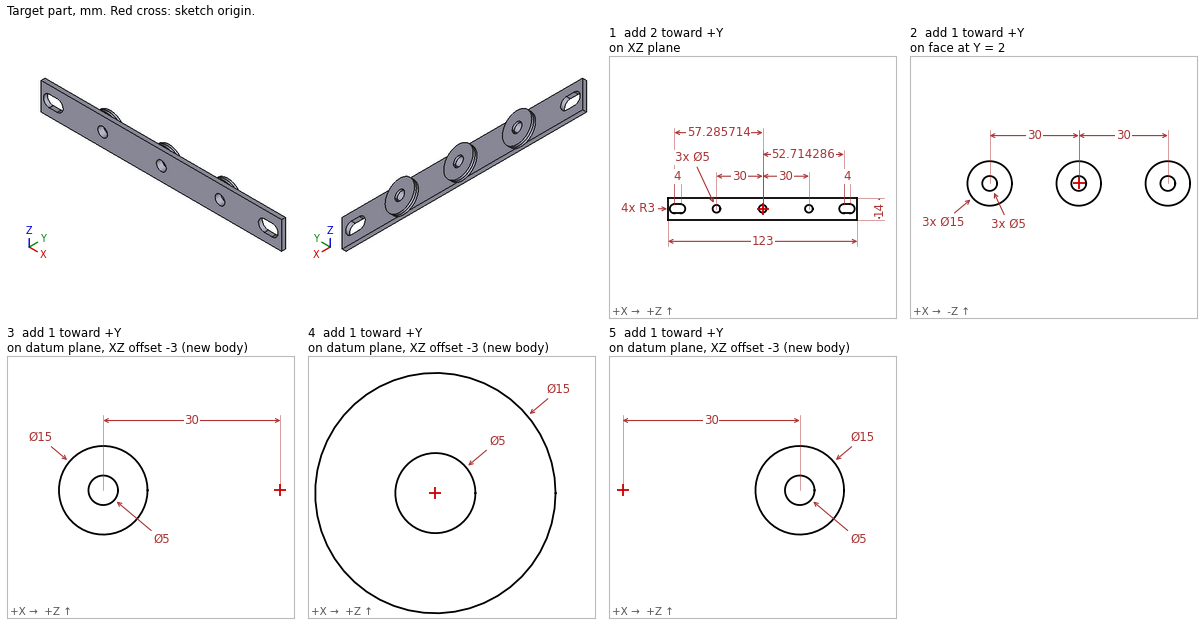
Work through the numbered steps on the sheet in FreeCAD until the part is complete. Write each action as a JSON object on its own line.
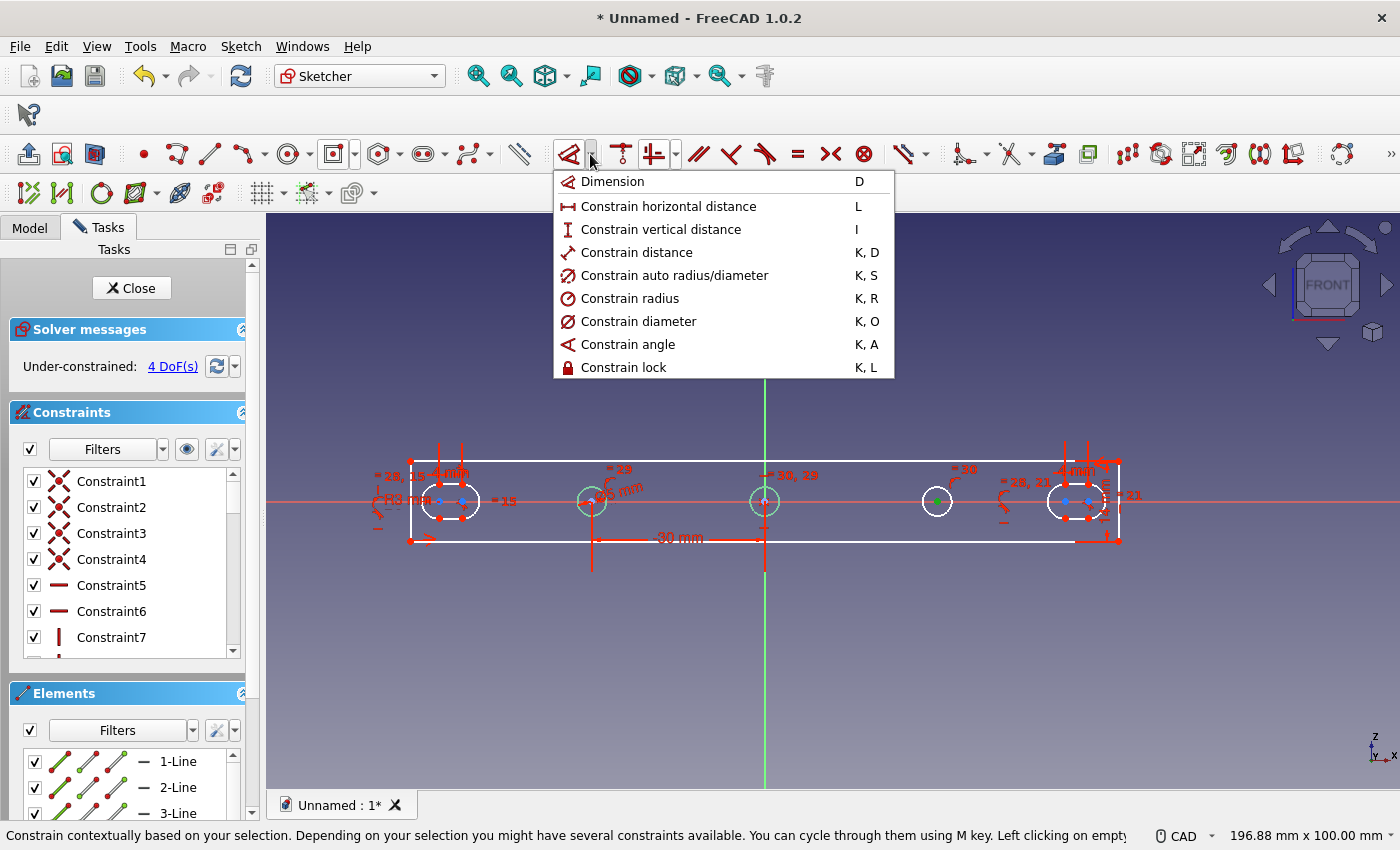
{"action": "left_click", "coordinate": [724, 206]}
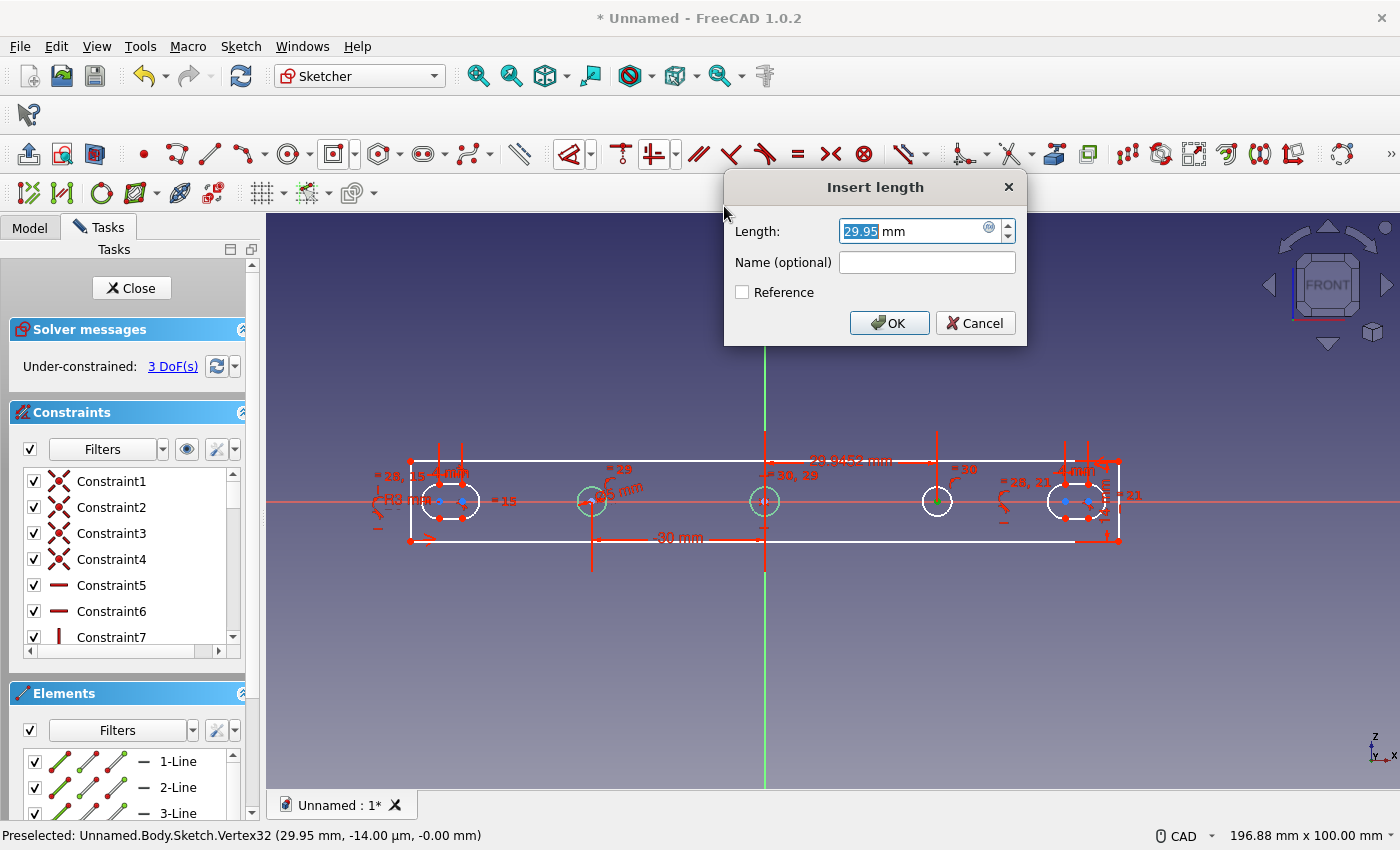
{"action": "type", "text": "30"}
{"action": "key", "text": "Return"}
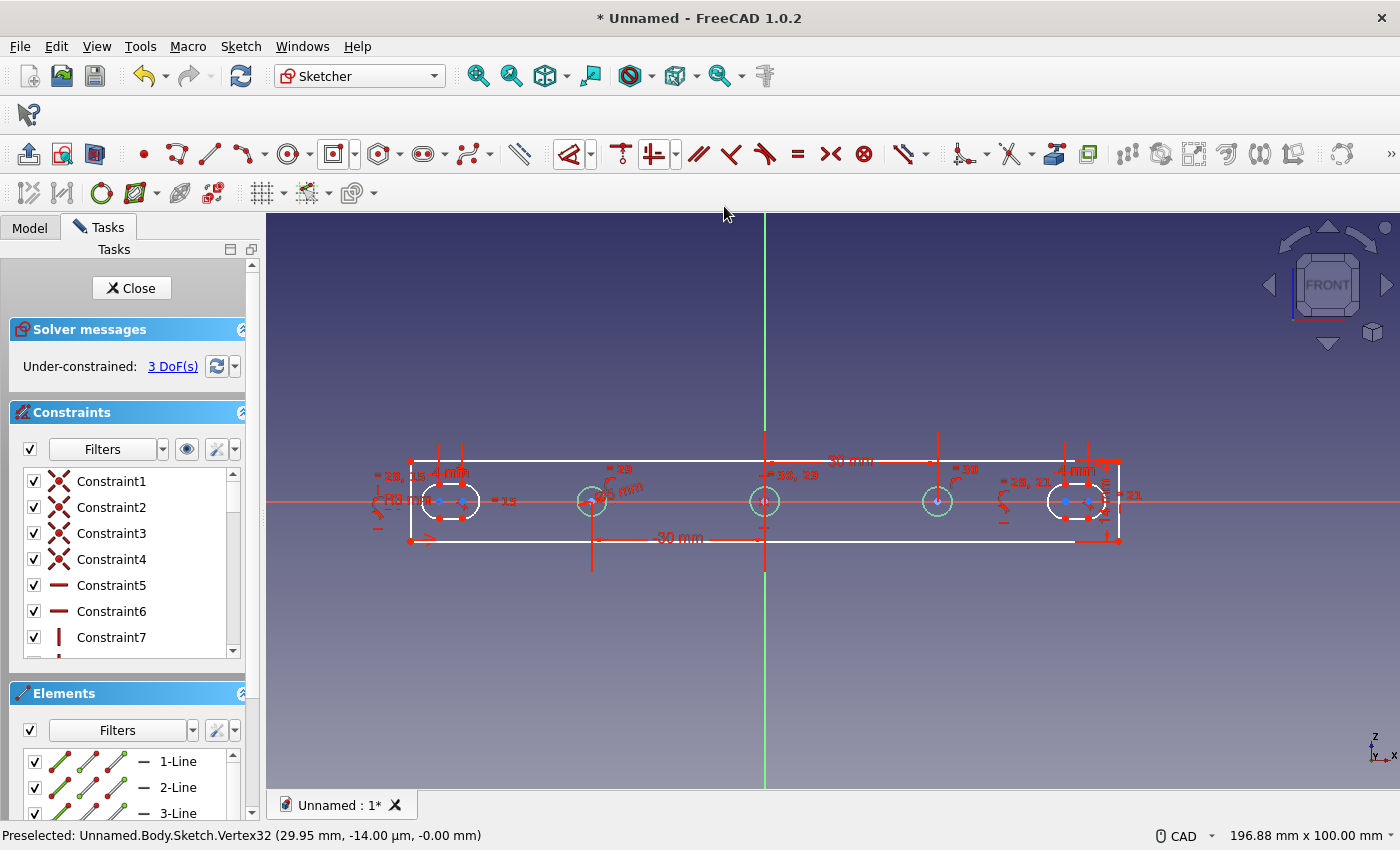
{"action": "left_click", "coordinate": [623, 542]}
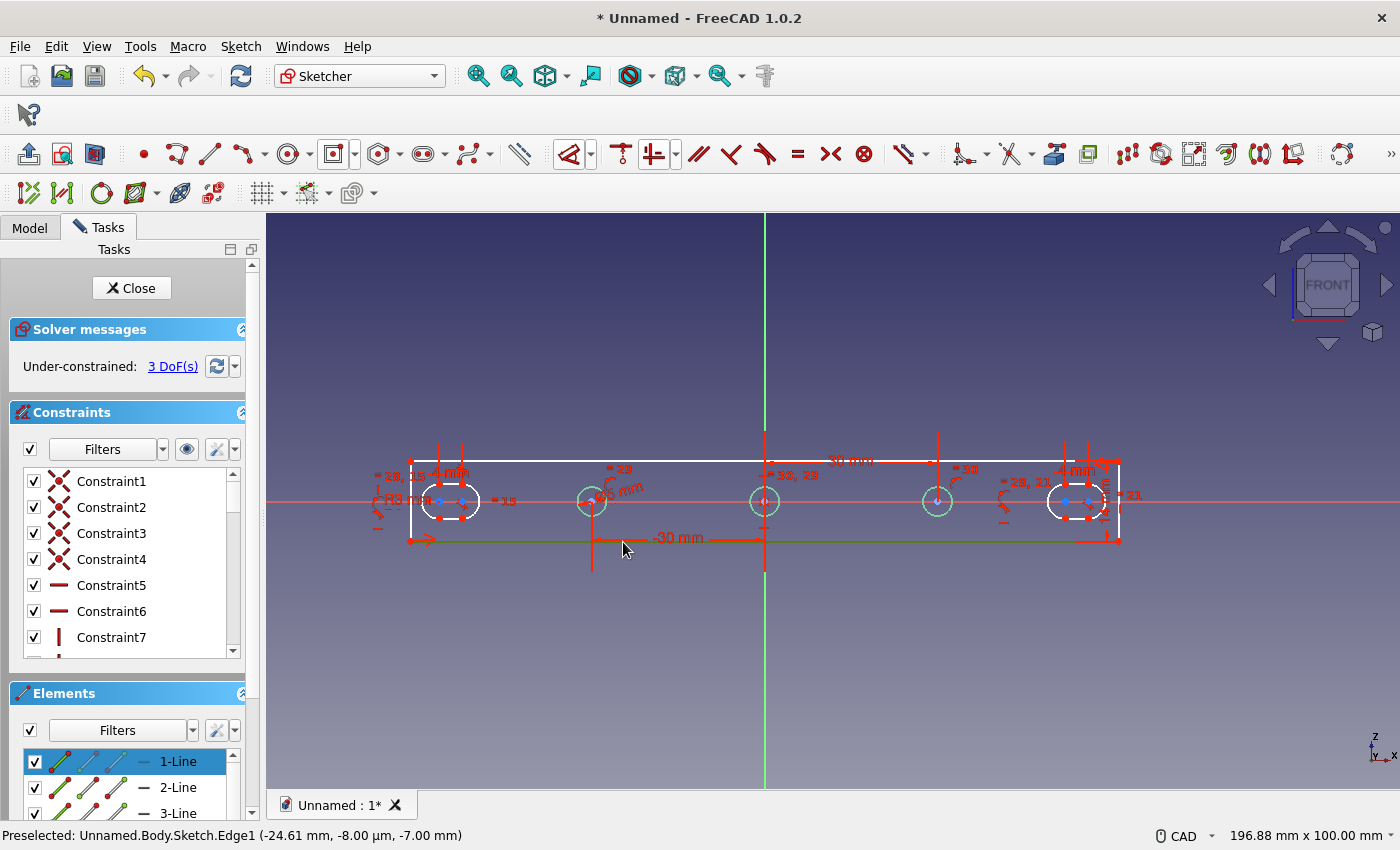
{"action": "left_click", "coordinate": [590, 154]}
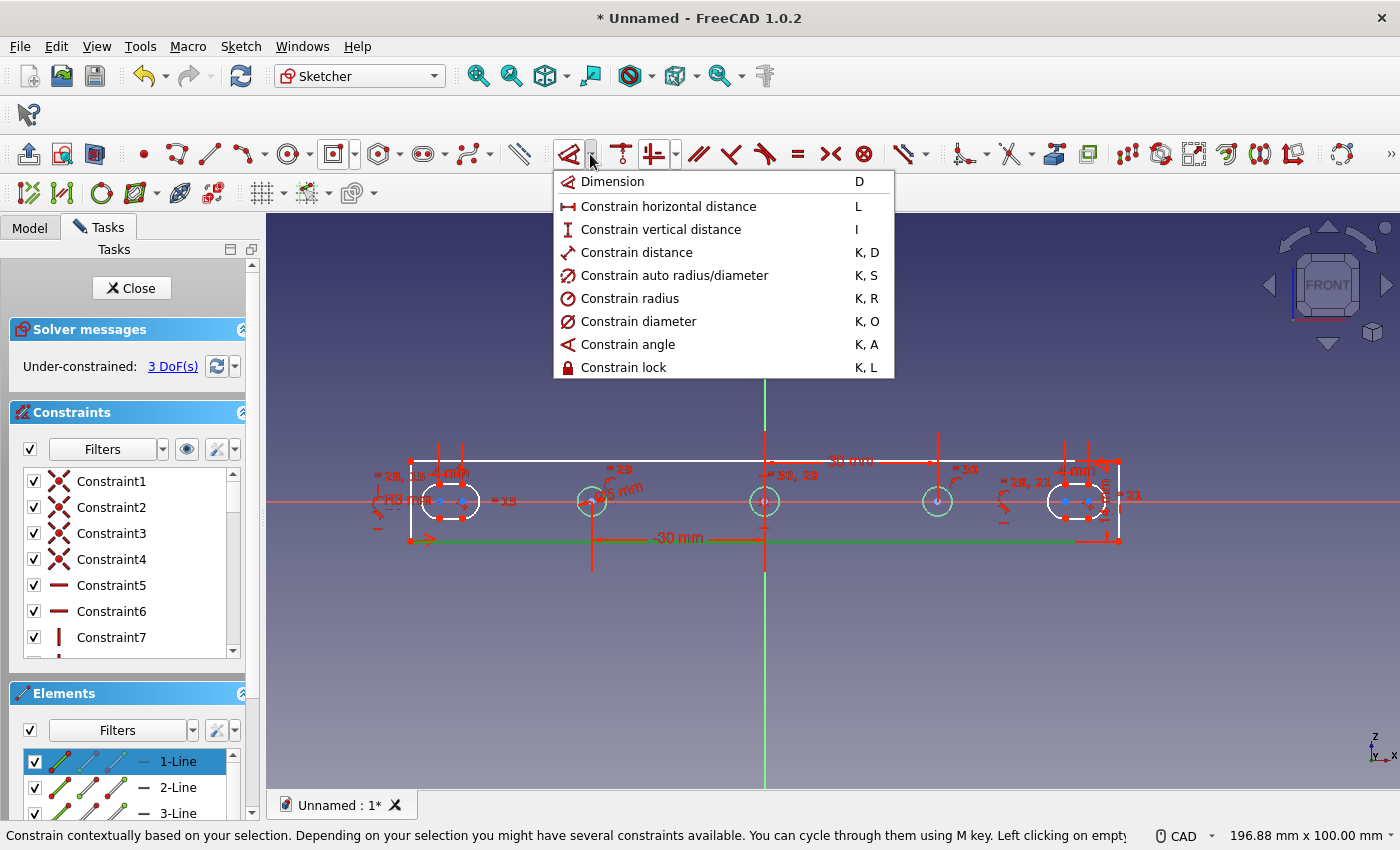
{"action": "left_click", "coordinate": [724, 206]}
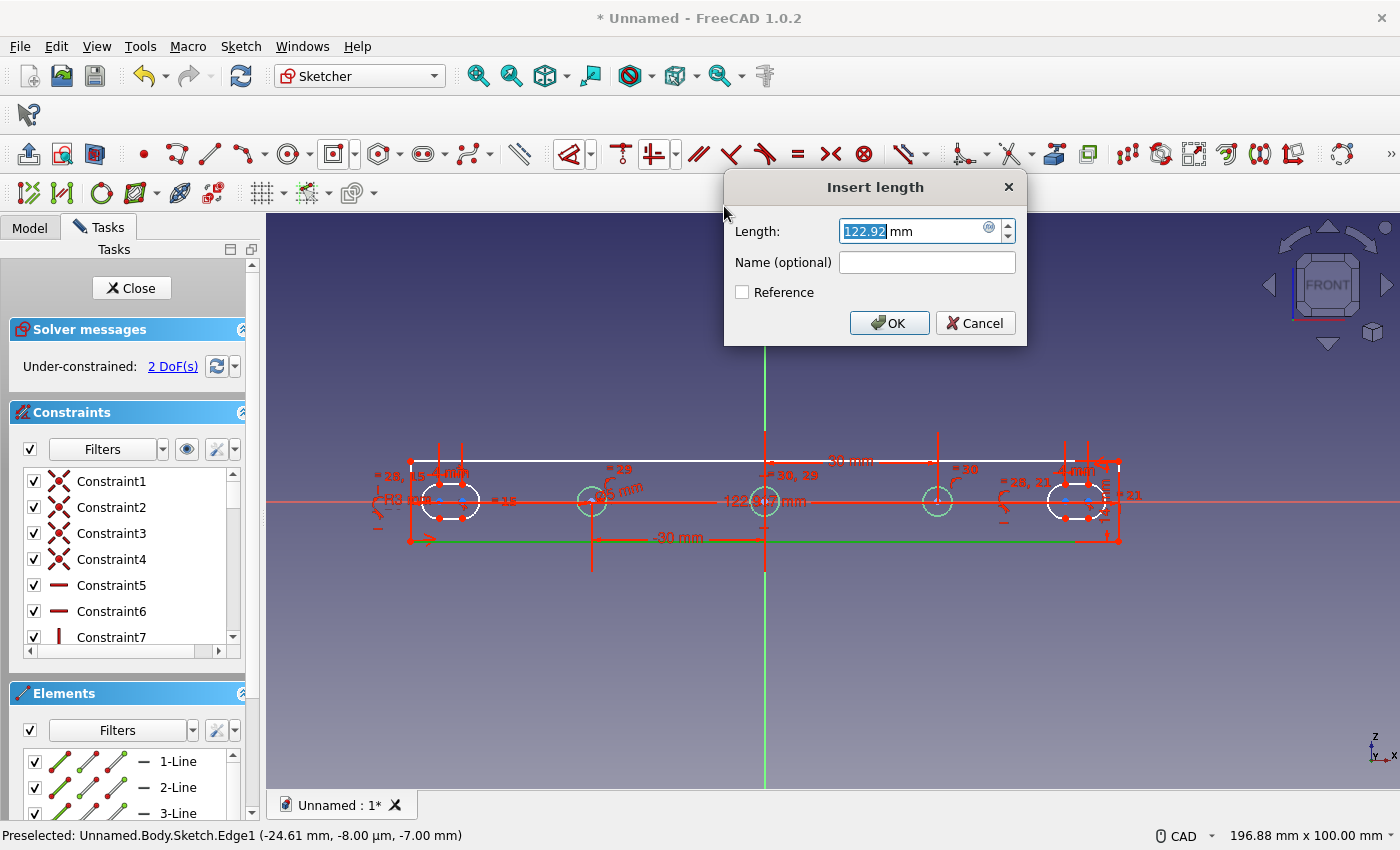
{"action": "type", "text": "123"}
{"action": "key", "text": "Return"}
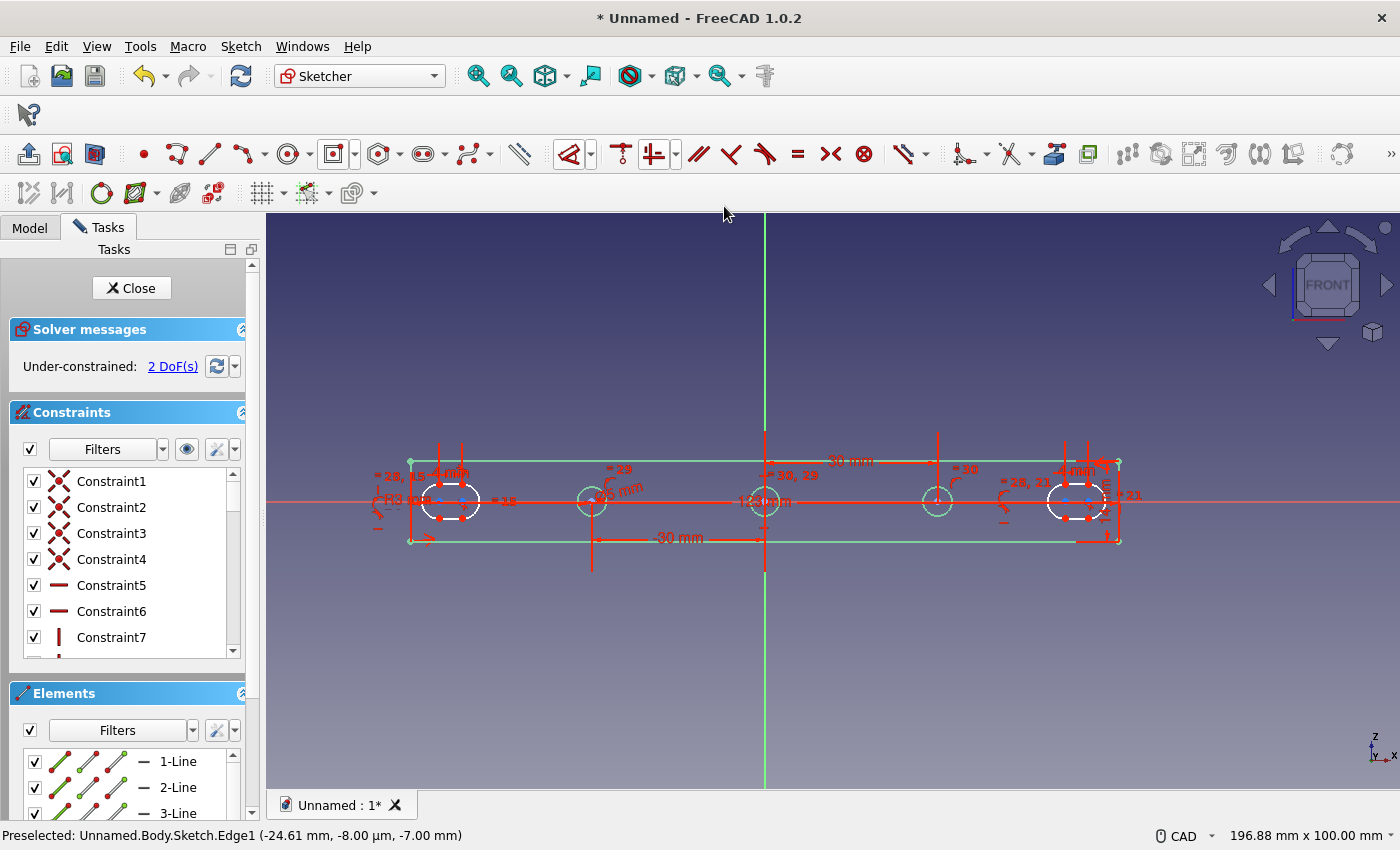
{"action": "left_click", "coordinate": [439, 484]}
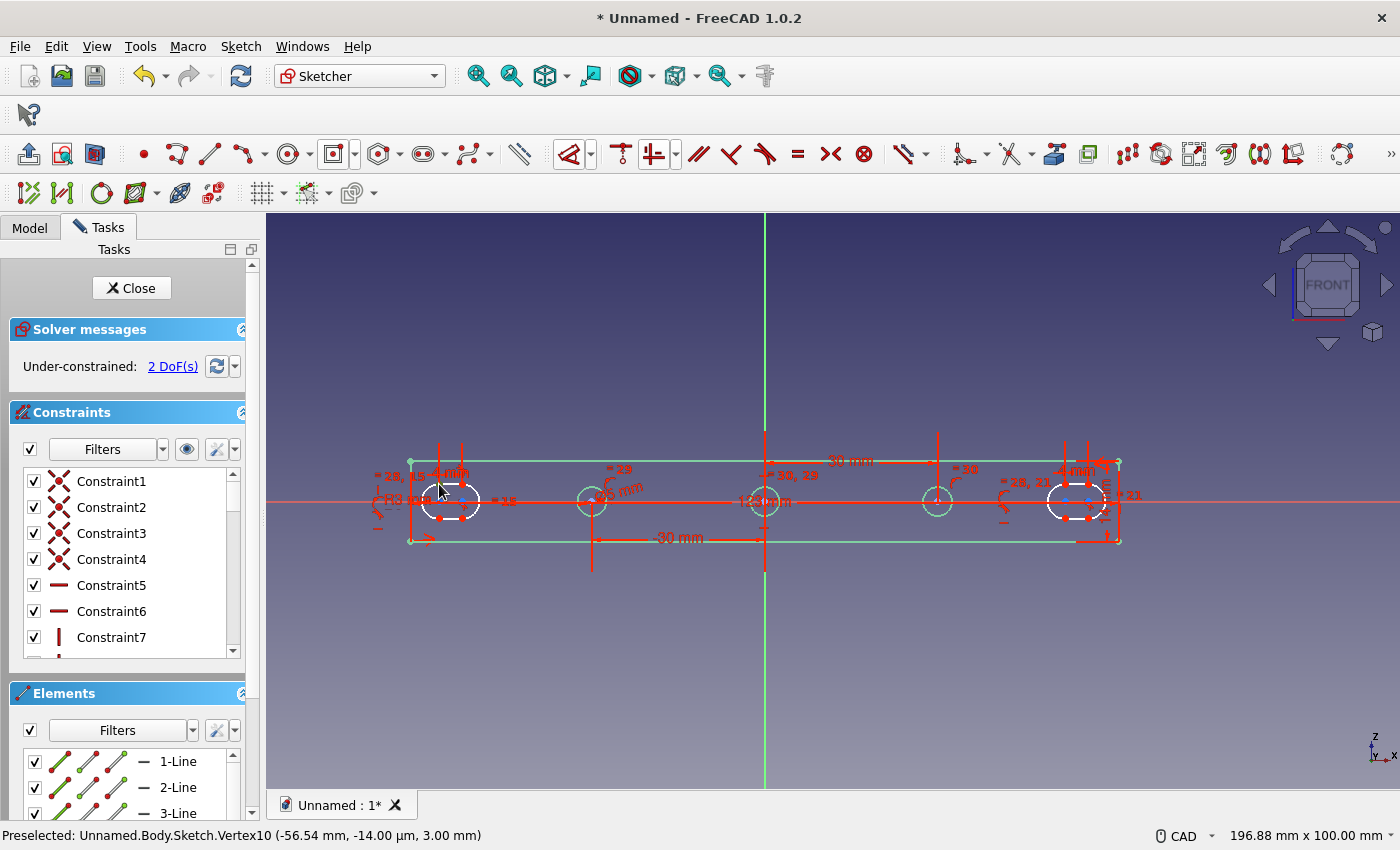
{"action": "key", "text": "l"}